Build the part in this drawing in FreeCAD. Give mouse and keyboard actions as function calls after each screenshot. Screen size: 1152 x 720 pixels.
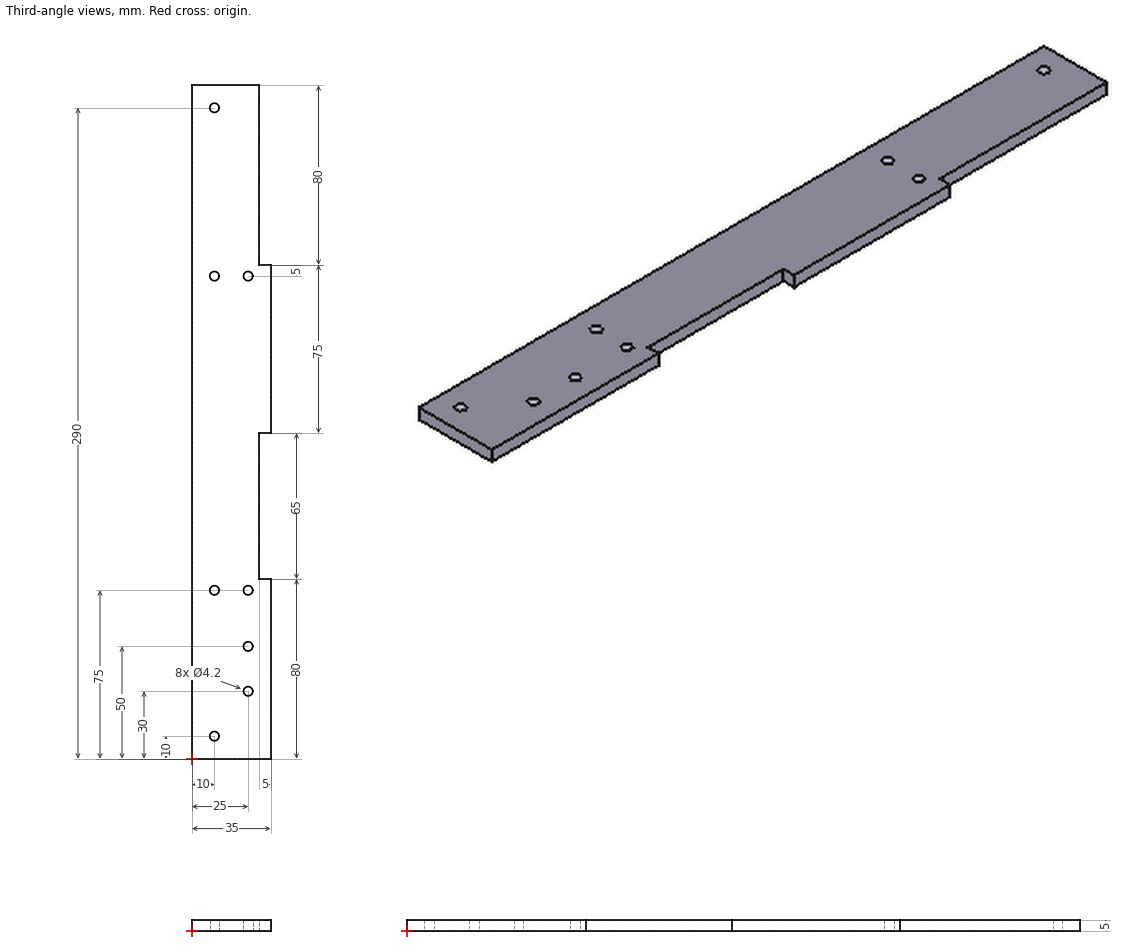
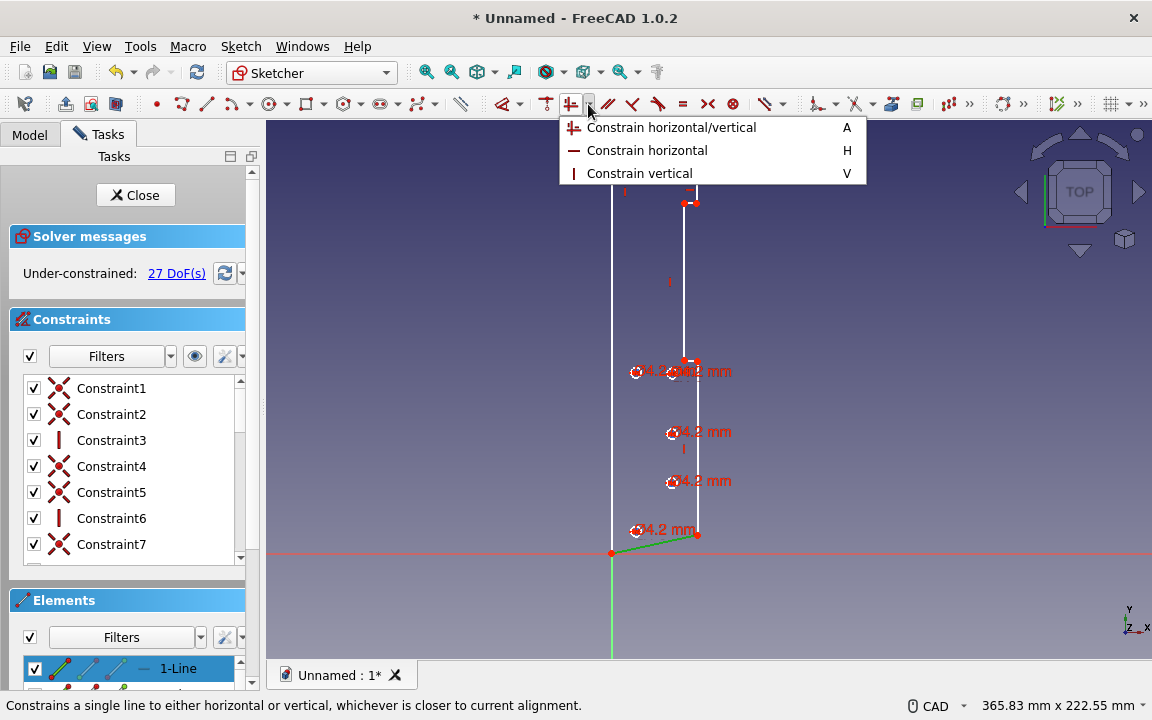
click(713, 150)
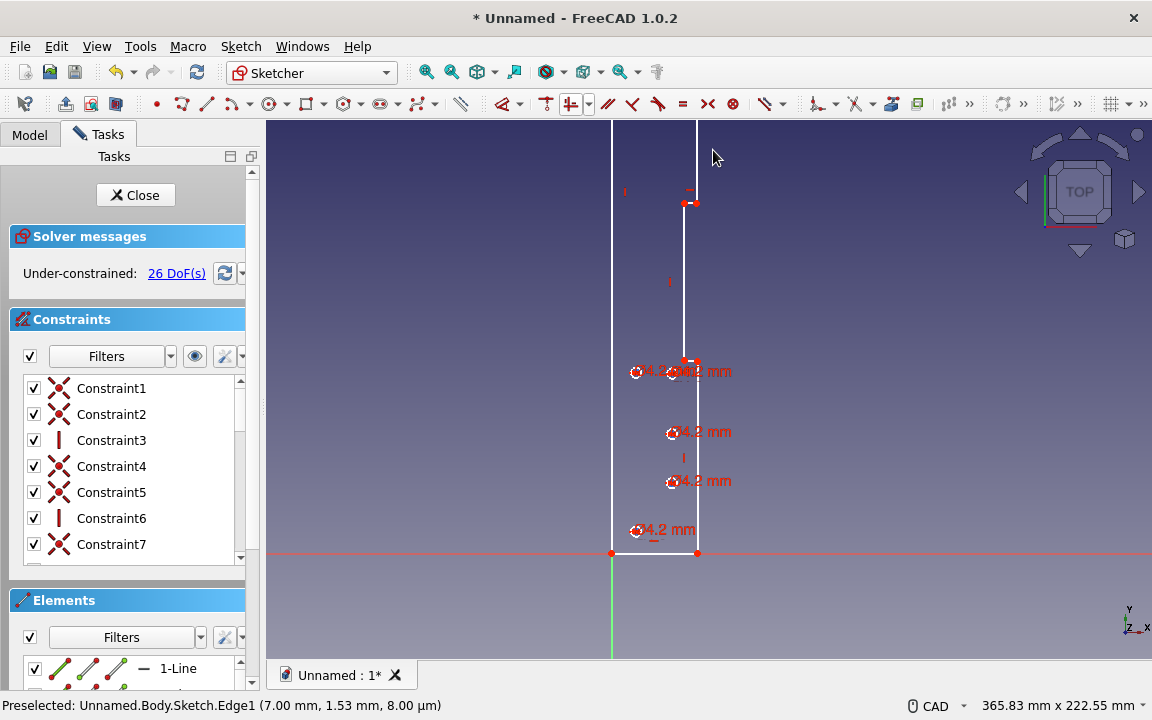
scroll(691, 361, up, 4)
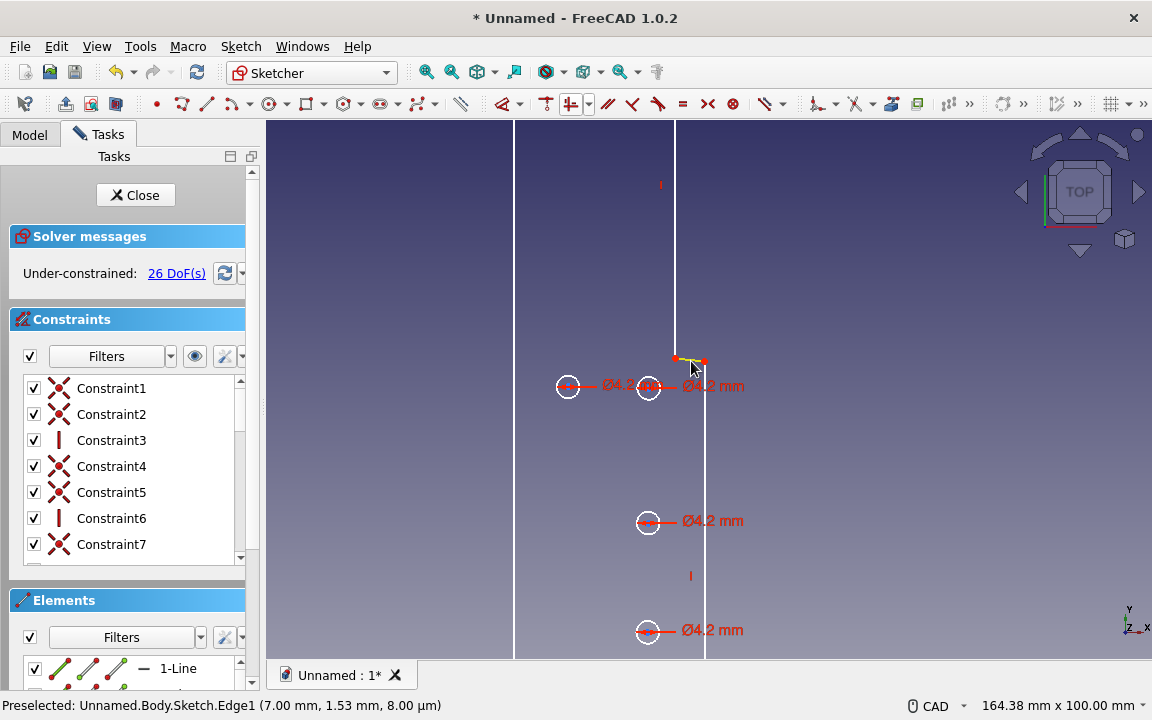
click(690, 360)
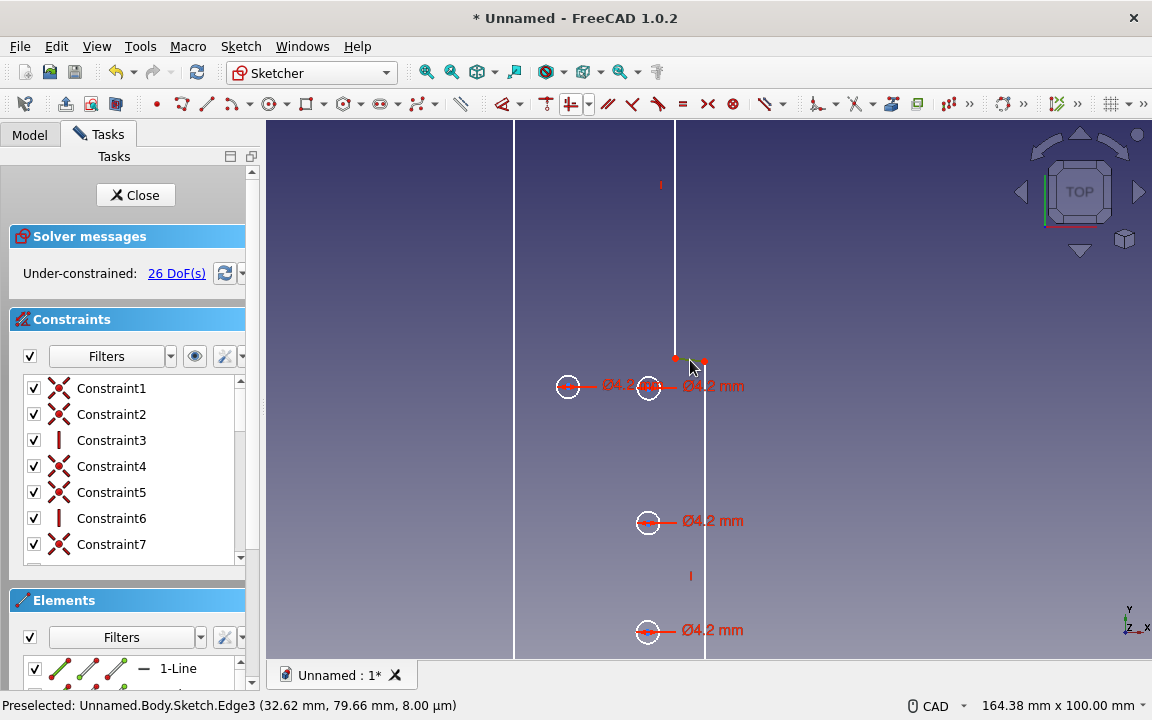
click(588, 104)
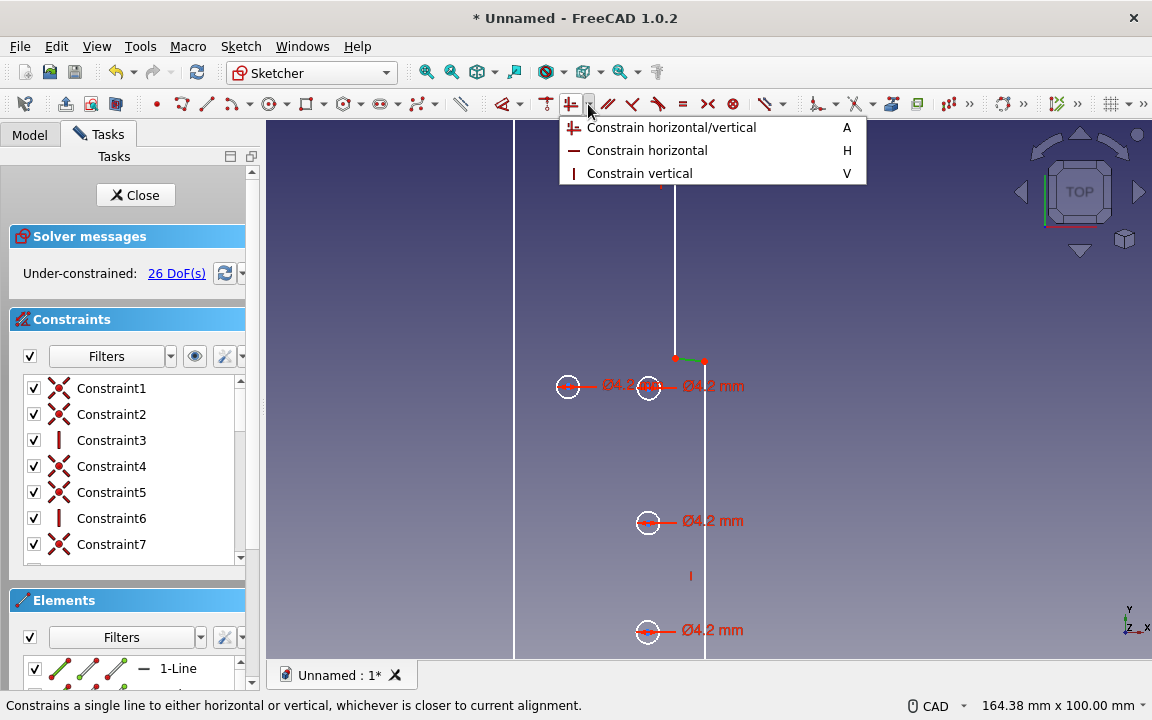
click(713, 150)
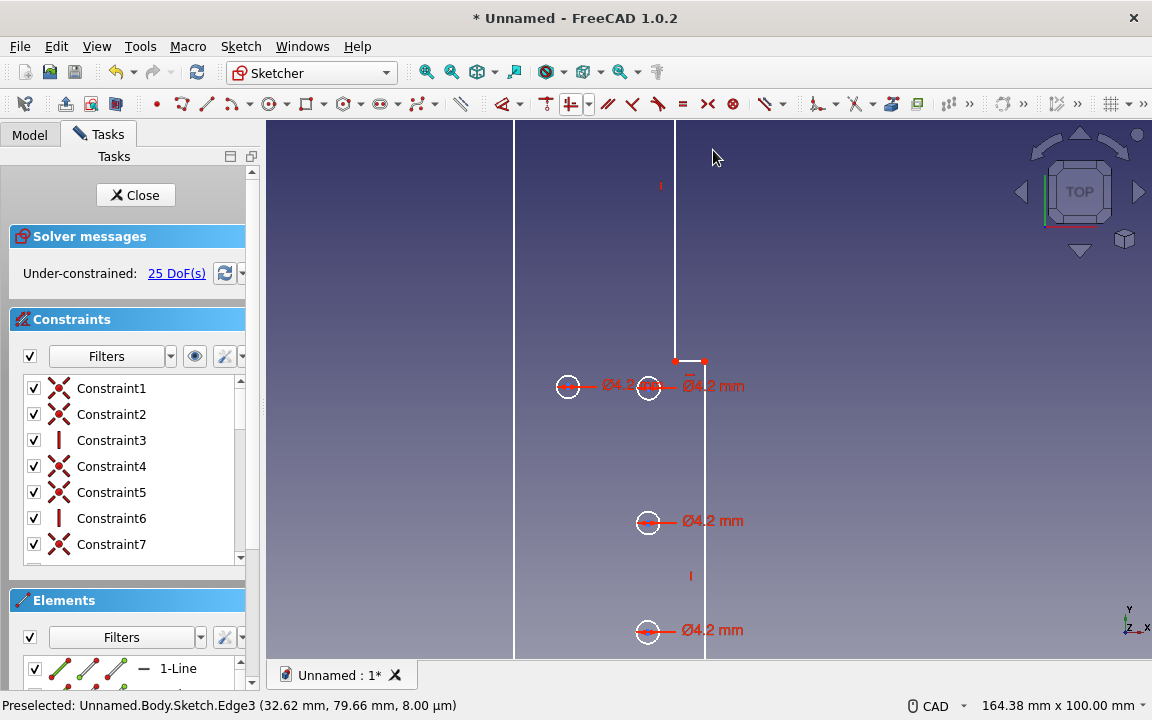
scroll(649, 493, down, 8)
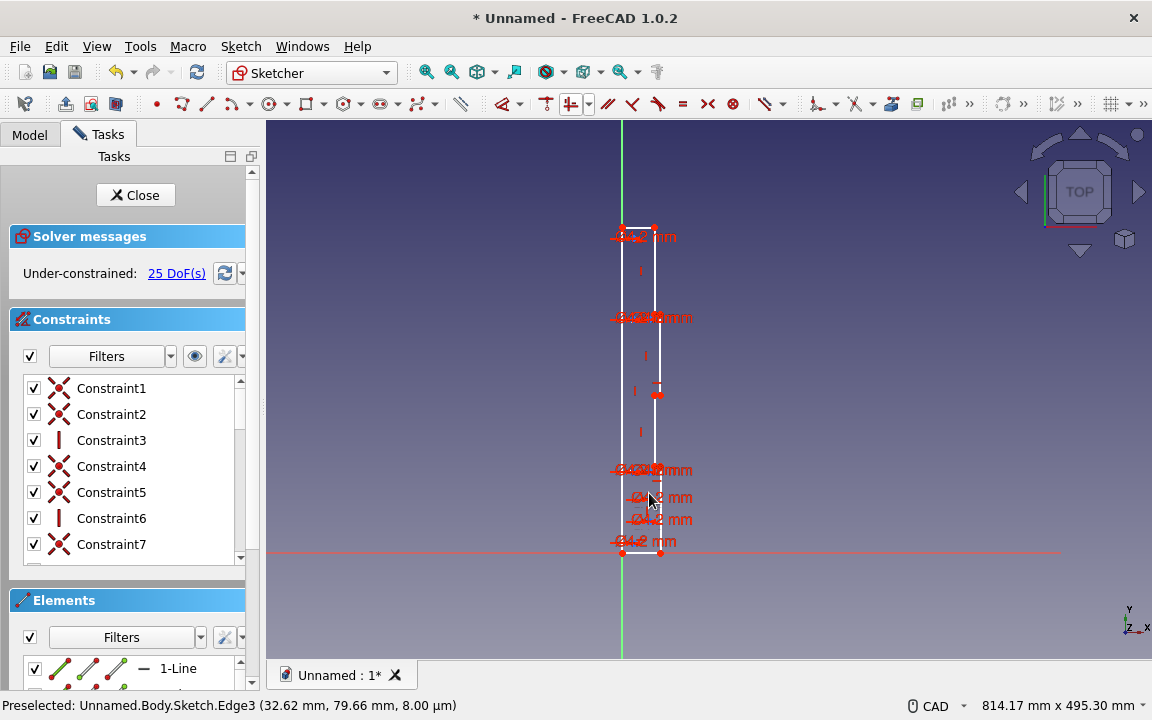
scroll(658, 315, up, 9)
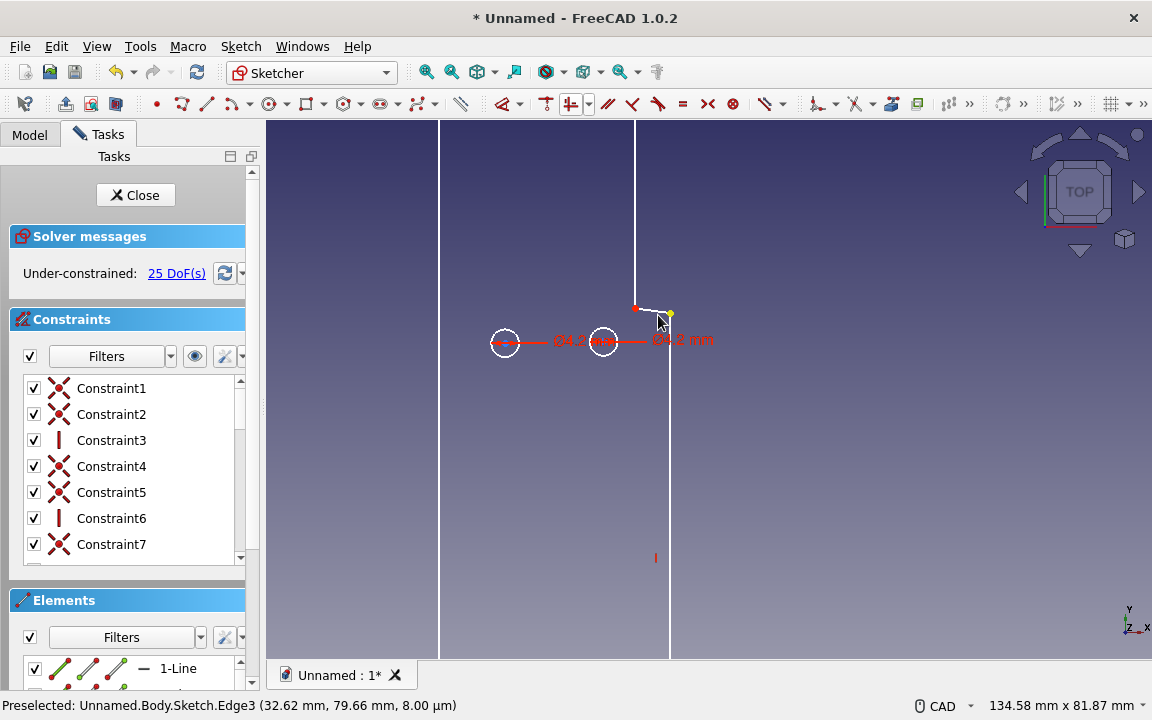
click(656, 311)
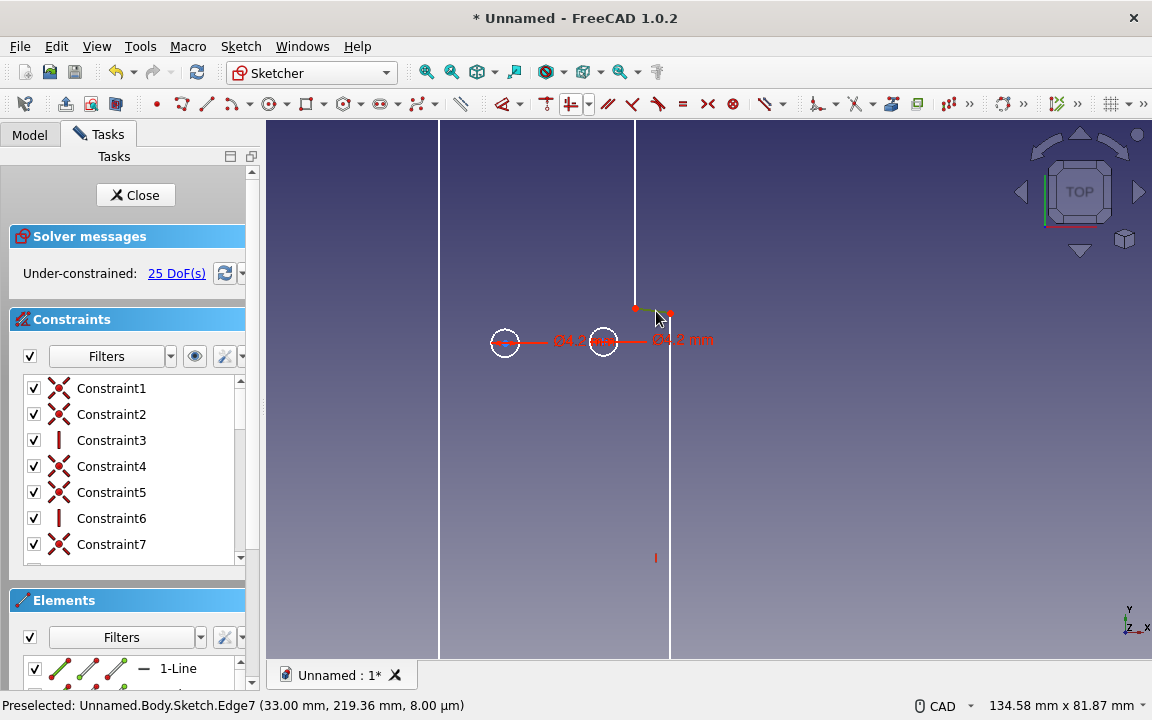
click(588, 104)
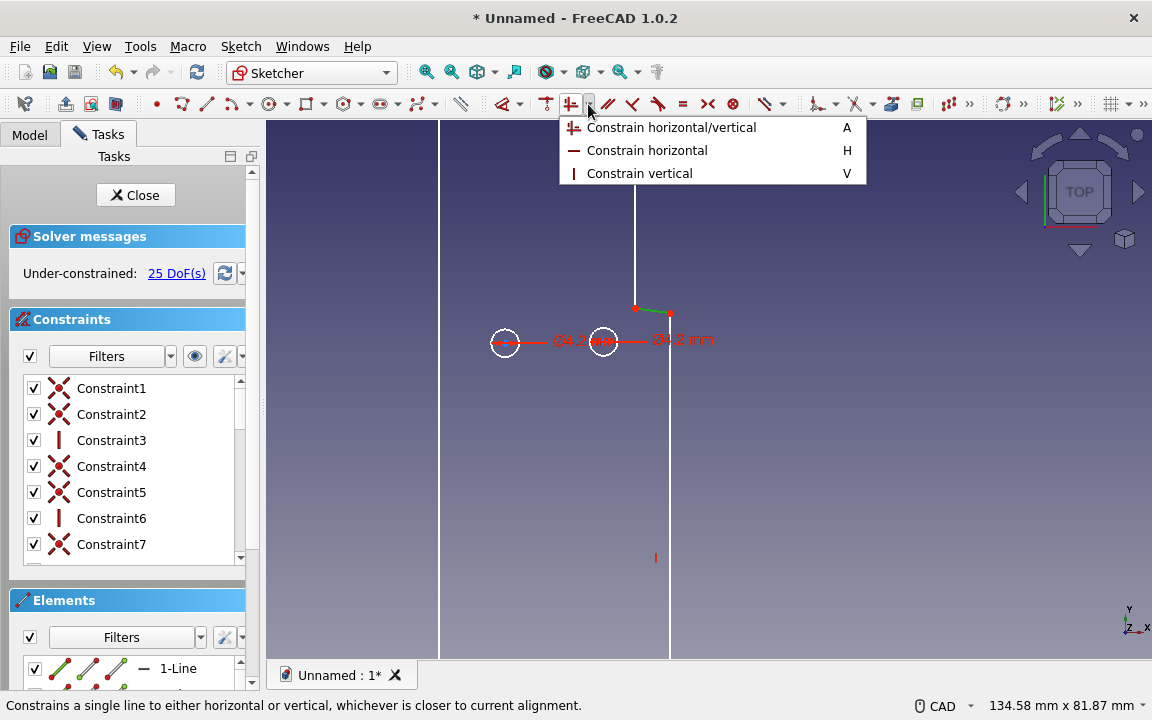
click(713, 150)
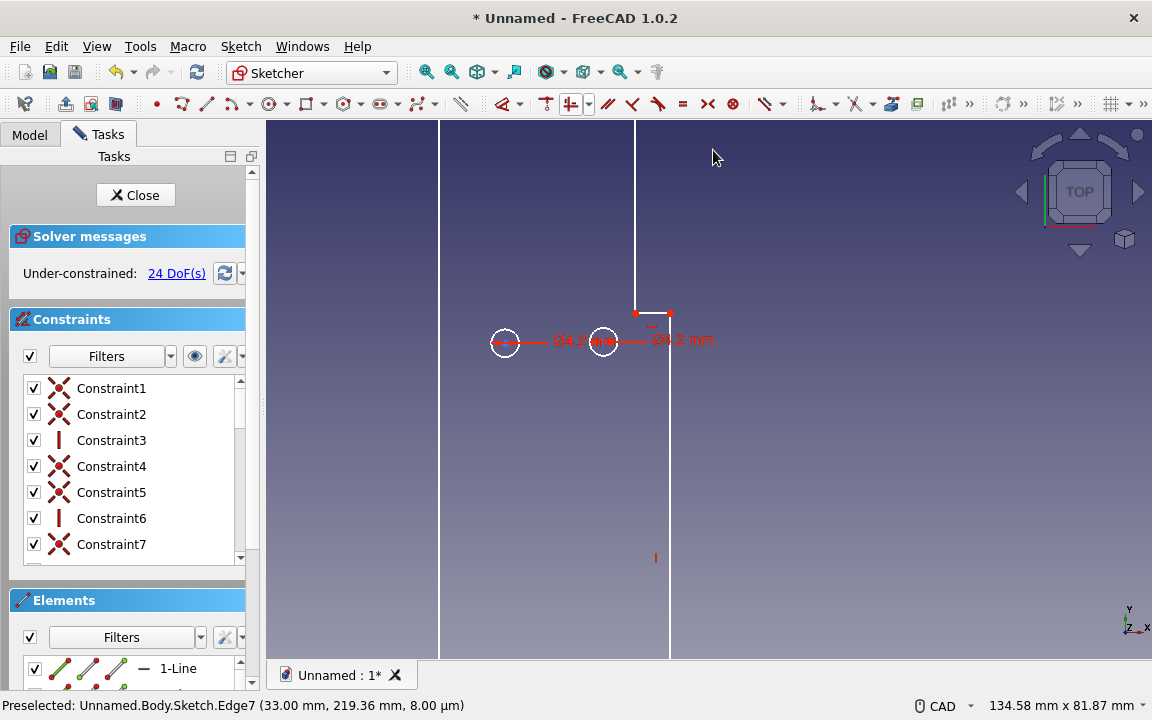
scroll(658, 315, down, 9)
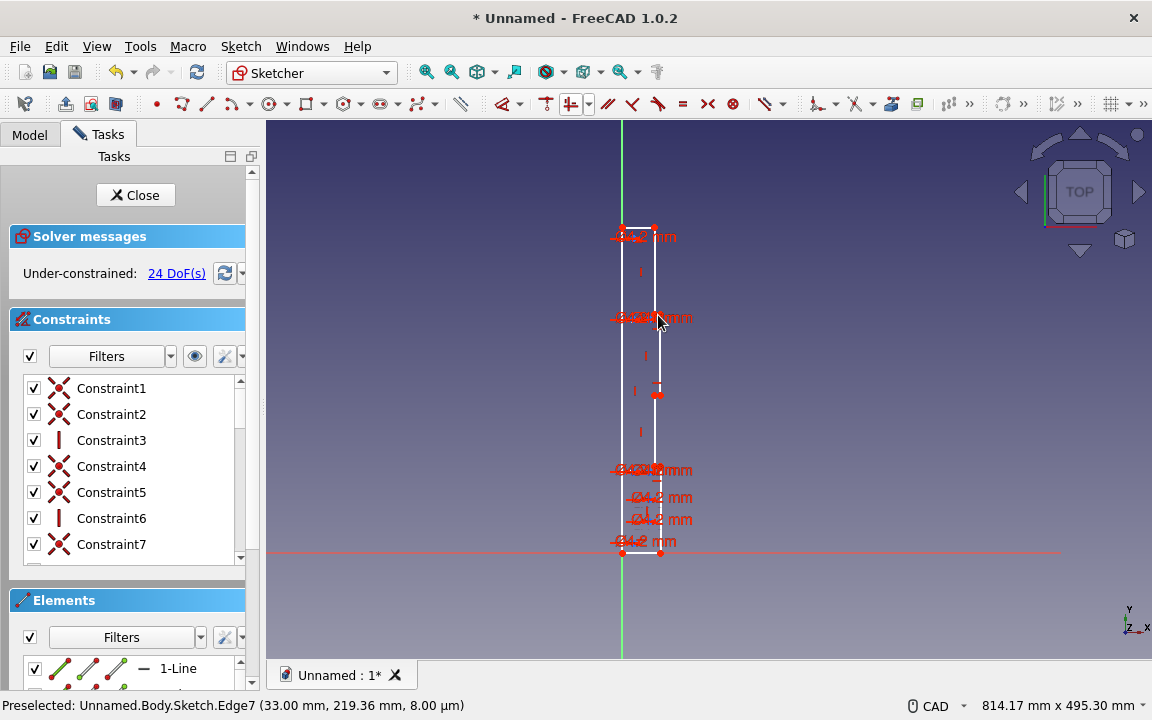
click(649, 522)